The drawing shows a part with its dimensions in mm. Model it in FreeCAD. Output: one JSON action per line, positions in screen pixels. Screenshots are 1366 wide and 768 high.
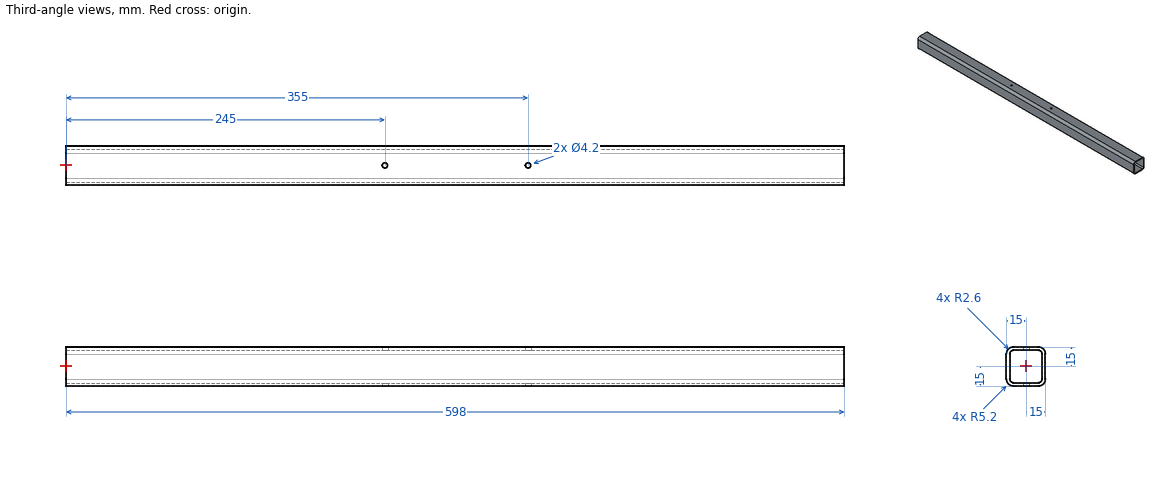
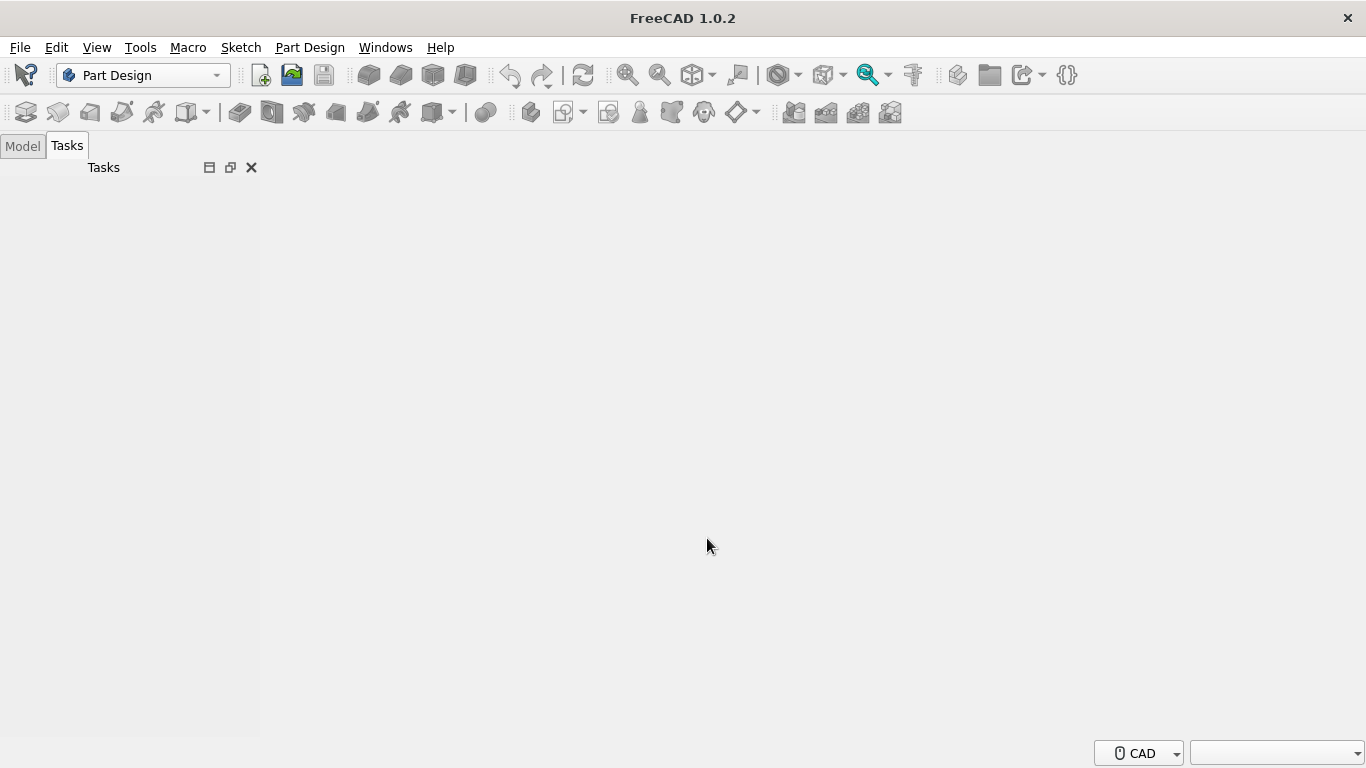
{"action": "left_click", "coordinate": [260, 76]}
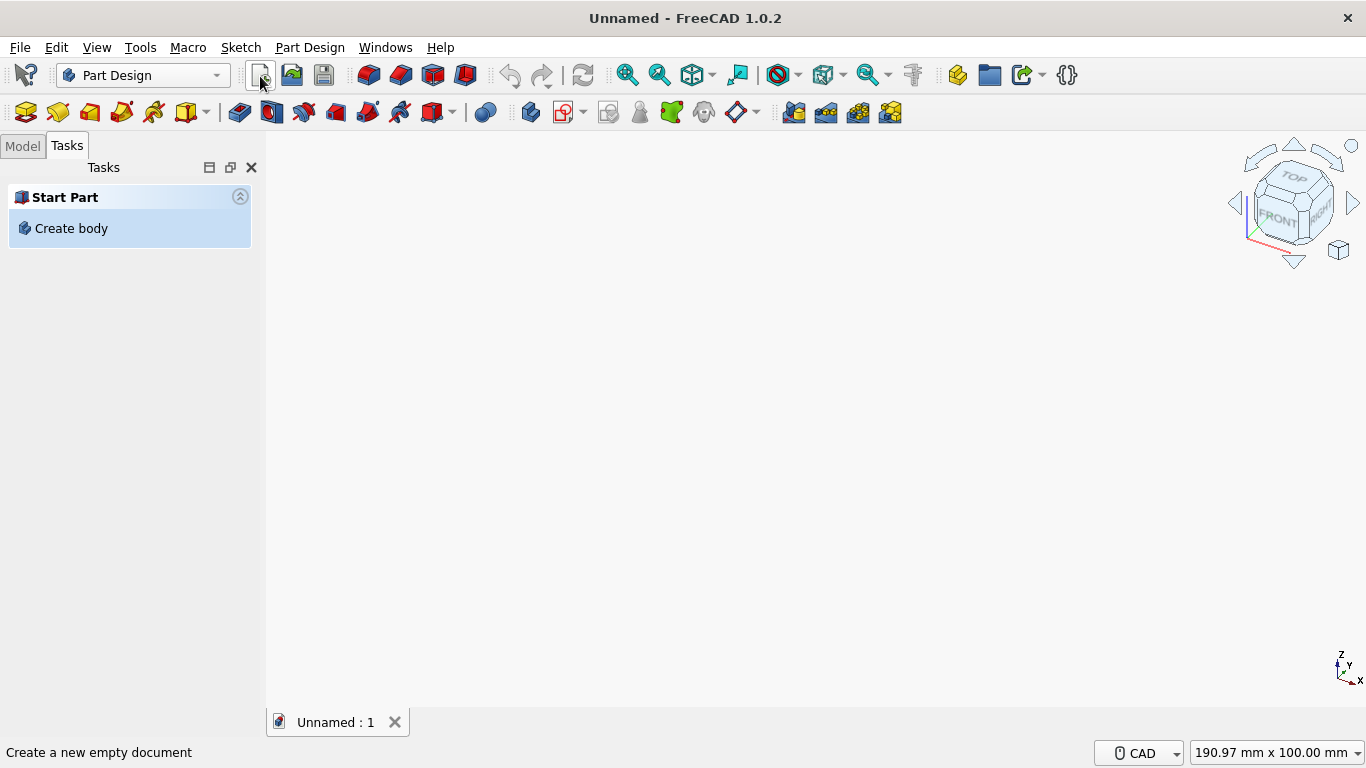
{"action": "left_click", "coordinate": [564, 112]}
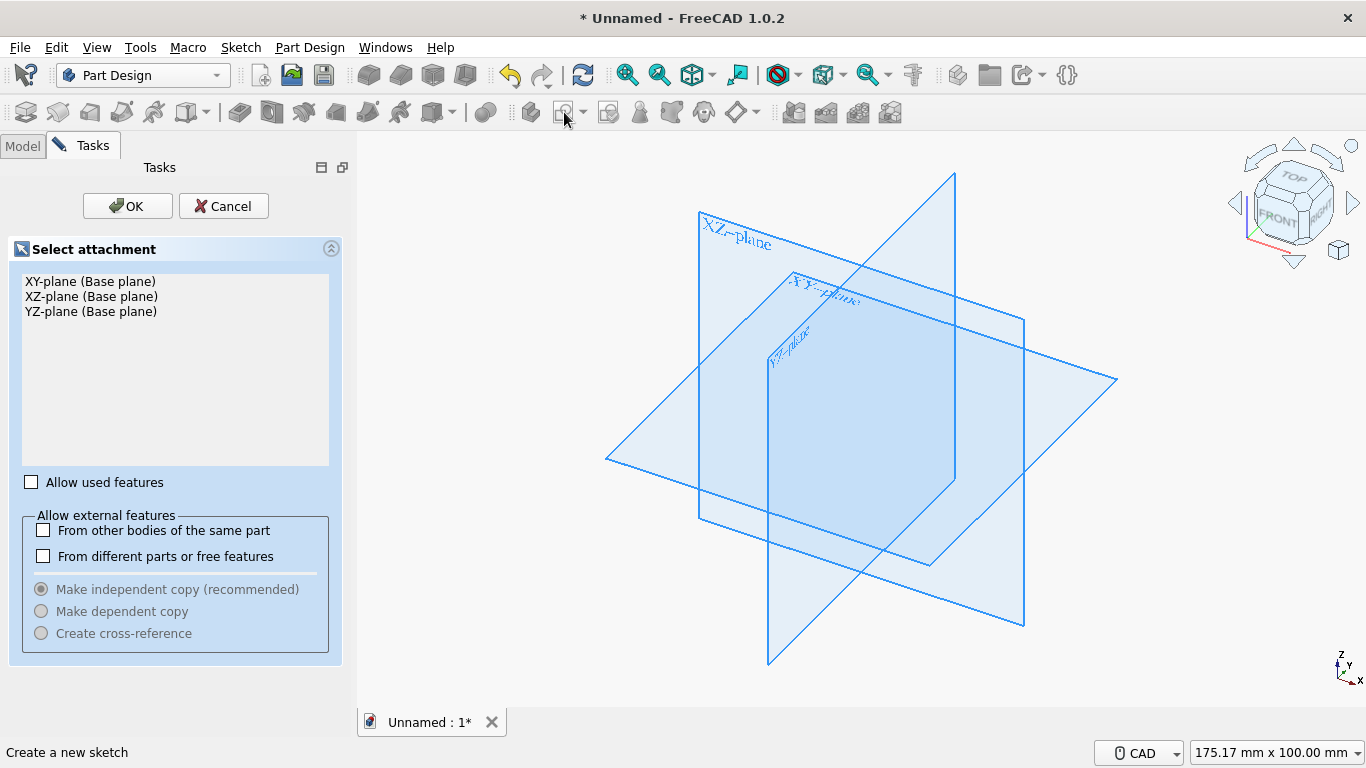
{"action": "left_click", "coordinate": [82, 312]}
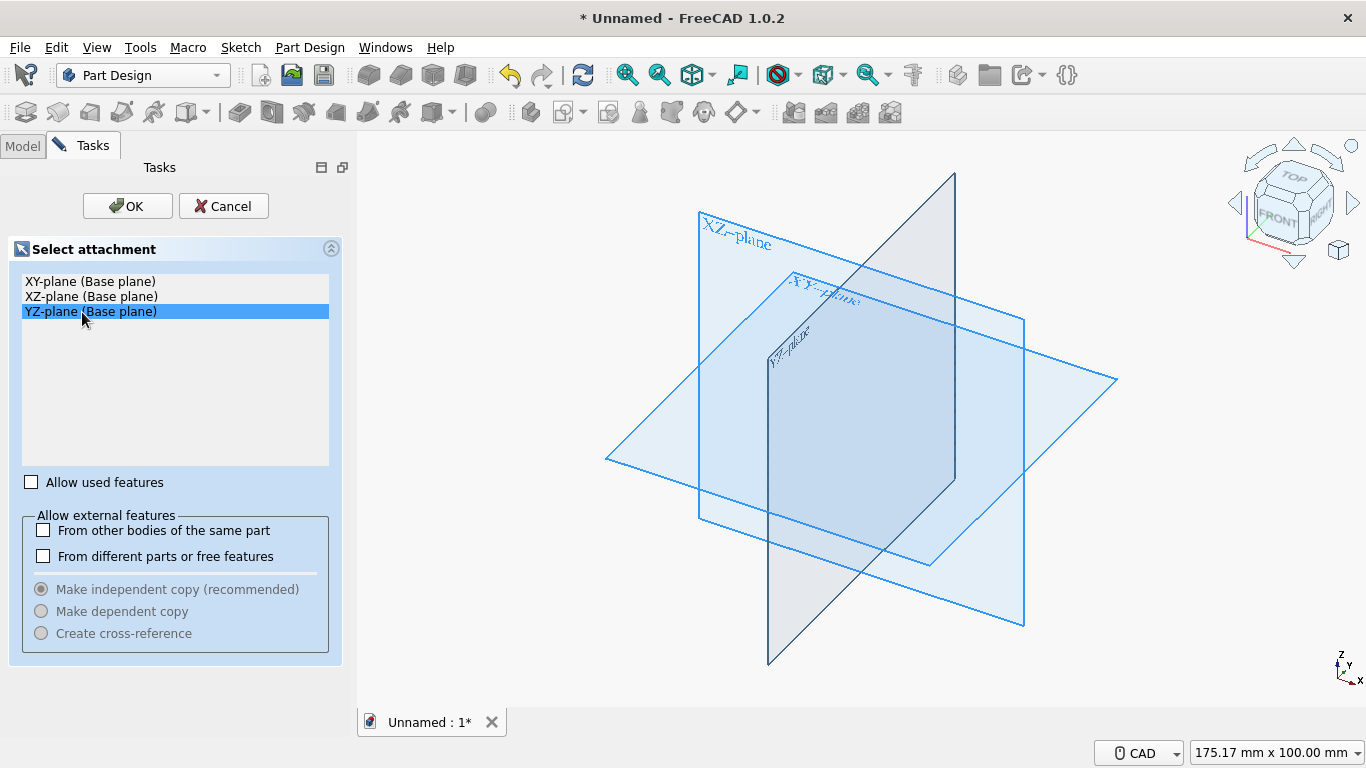
{"action": "left_click", "coordinate": [128, 206]}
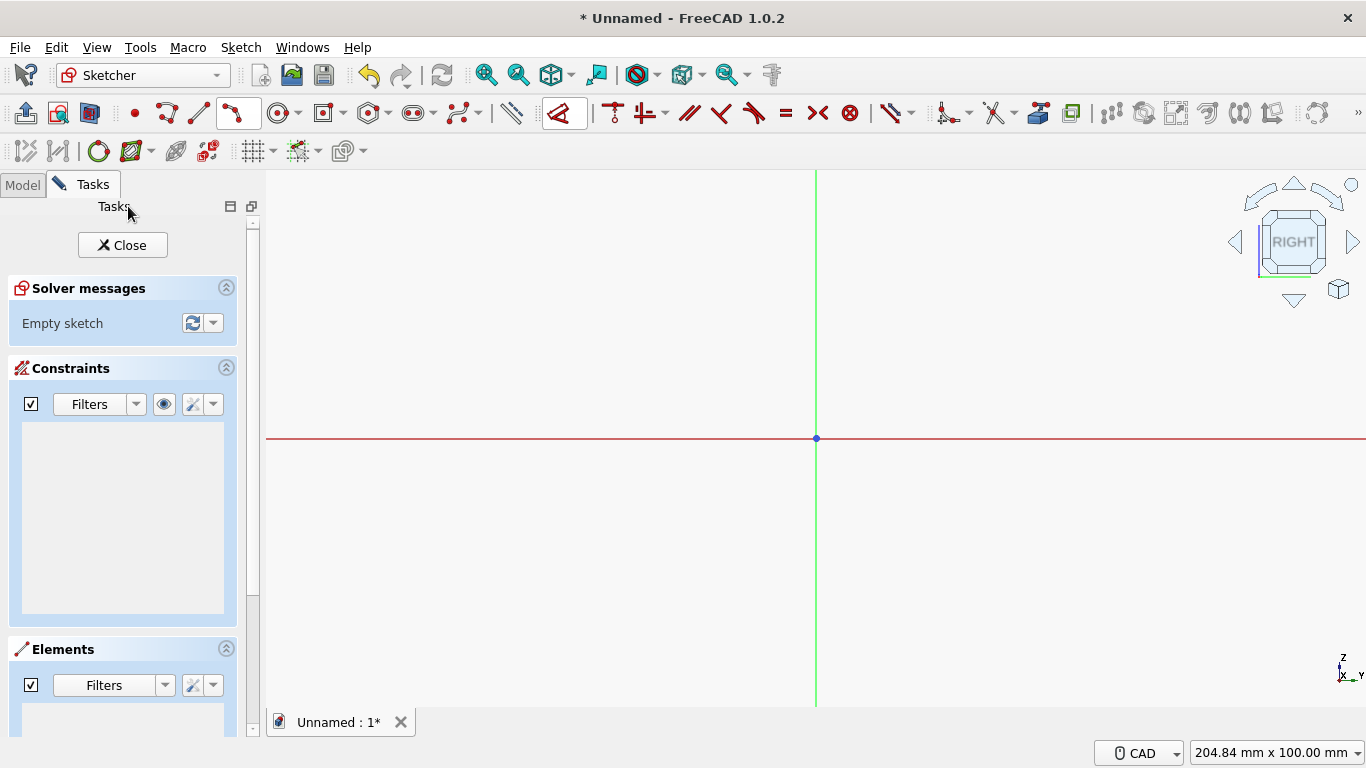
{"action": "scroll", "coordinate": [872, 438], "scroll_direction": "up", "scroll_amount": 4}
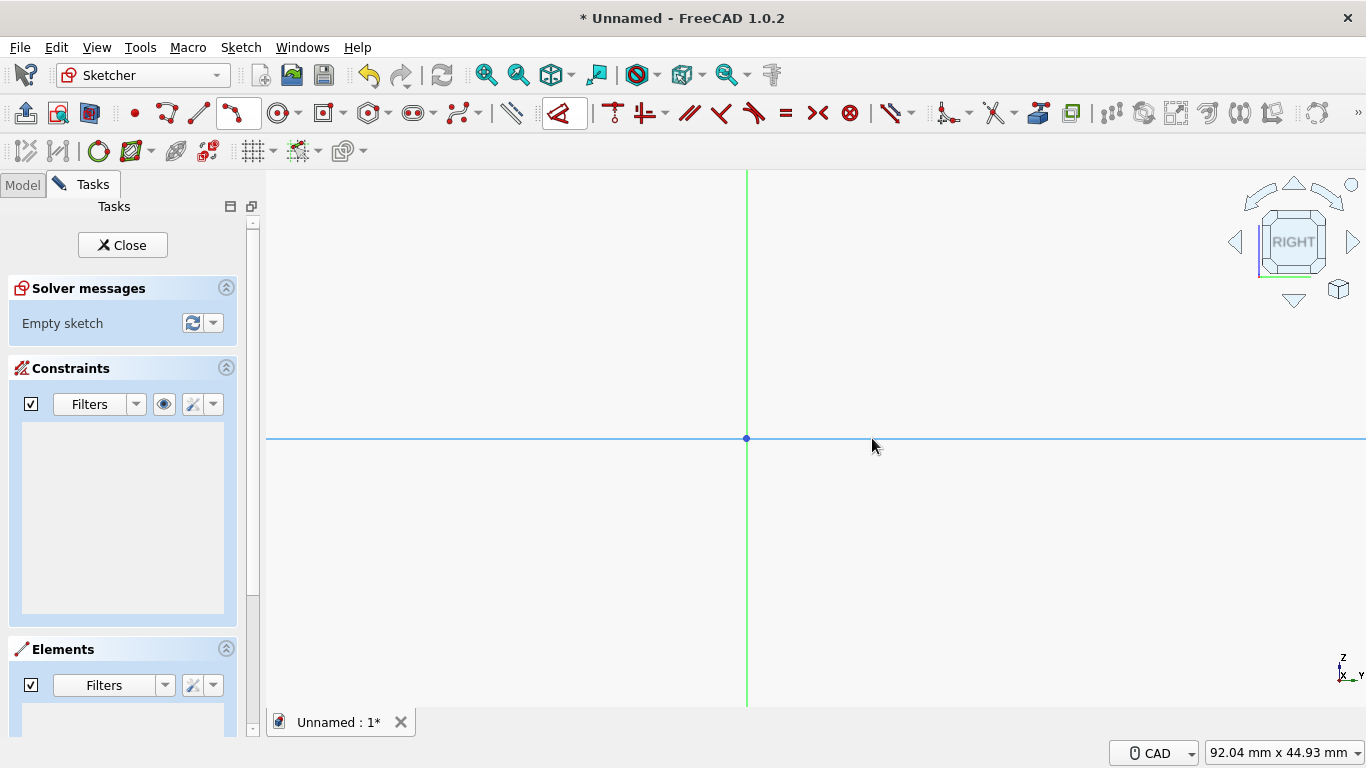
{"action": "key", "text": "g l"}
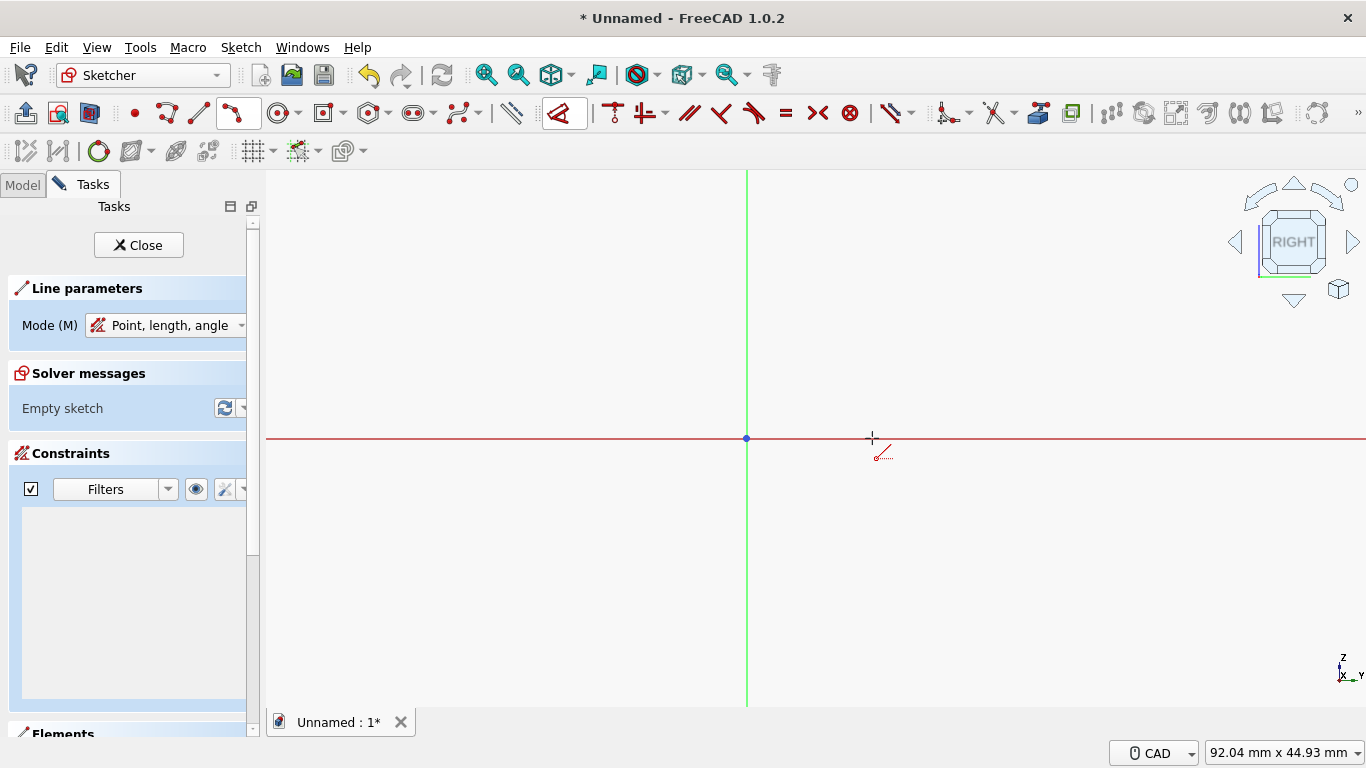
{"action": "left_click", "coordinate": [567, 321]}
{"action": "left_click", "coordinate": [567, 556]}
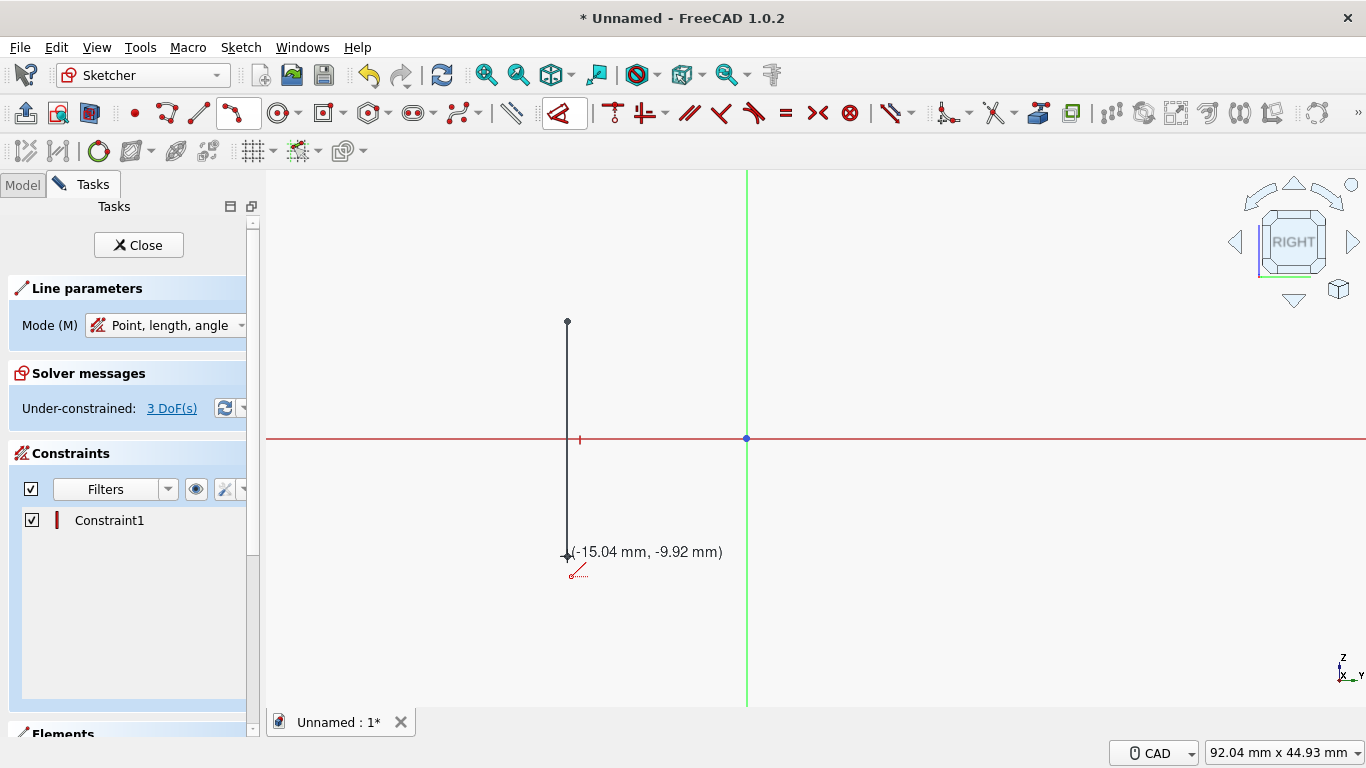
{"action": "left_click", "coordinate": [630, 618]}
{"action": "left_click", "coordinate": [864, 618]}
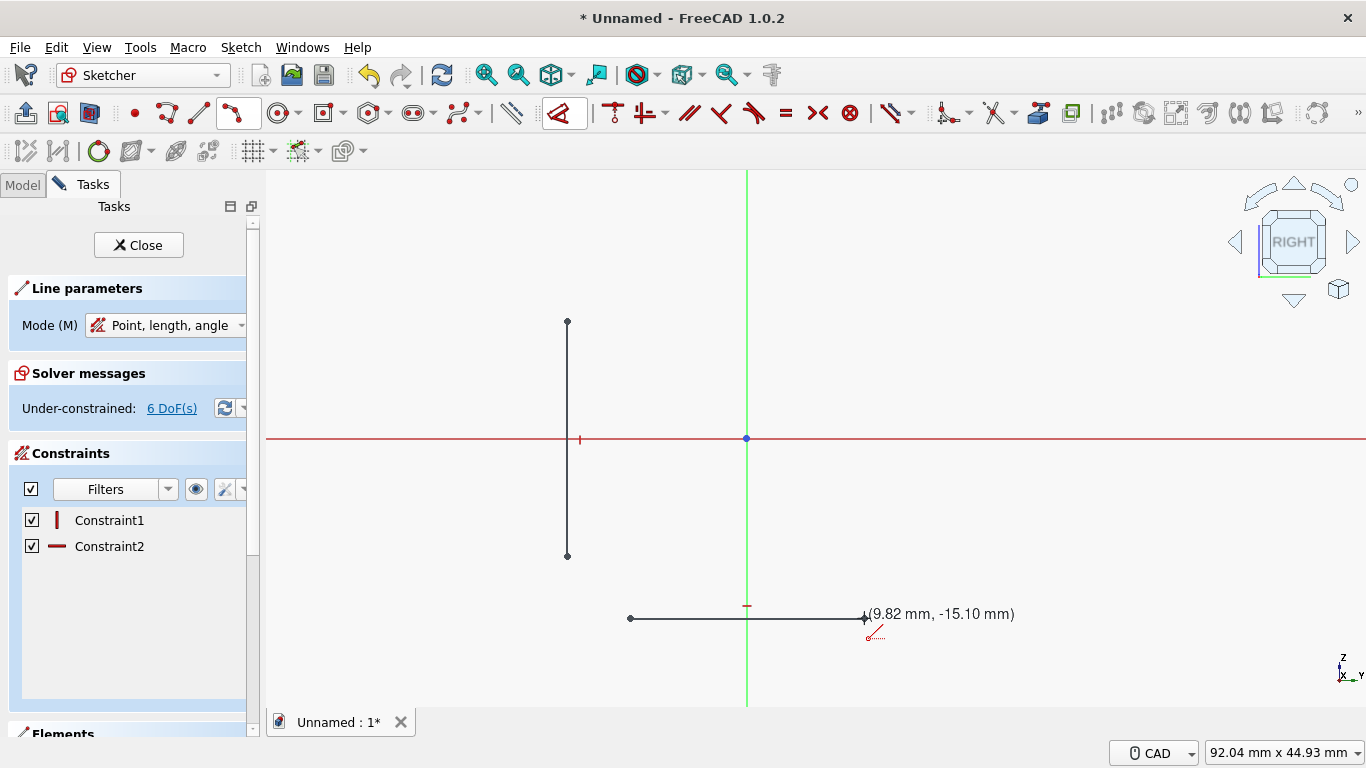
{"action": "left_click", "coordinate": [926, 556]}
{"action": "left_click", "coordinate": [926, 321]}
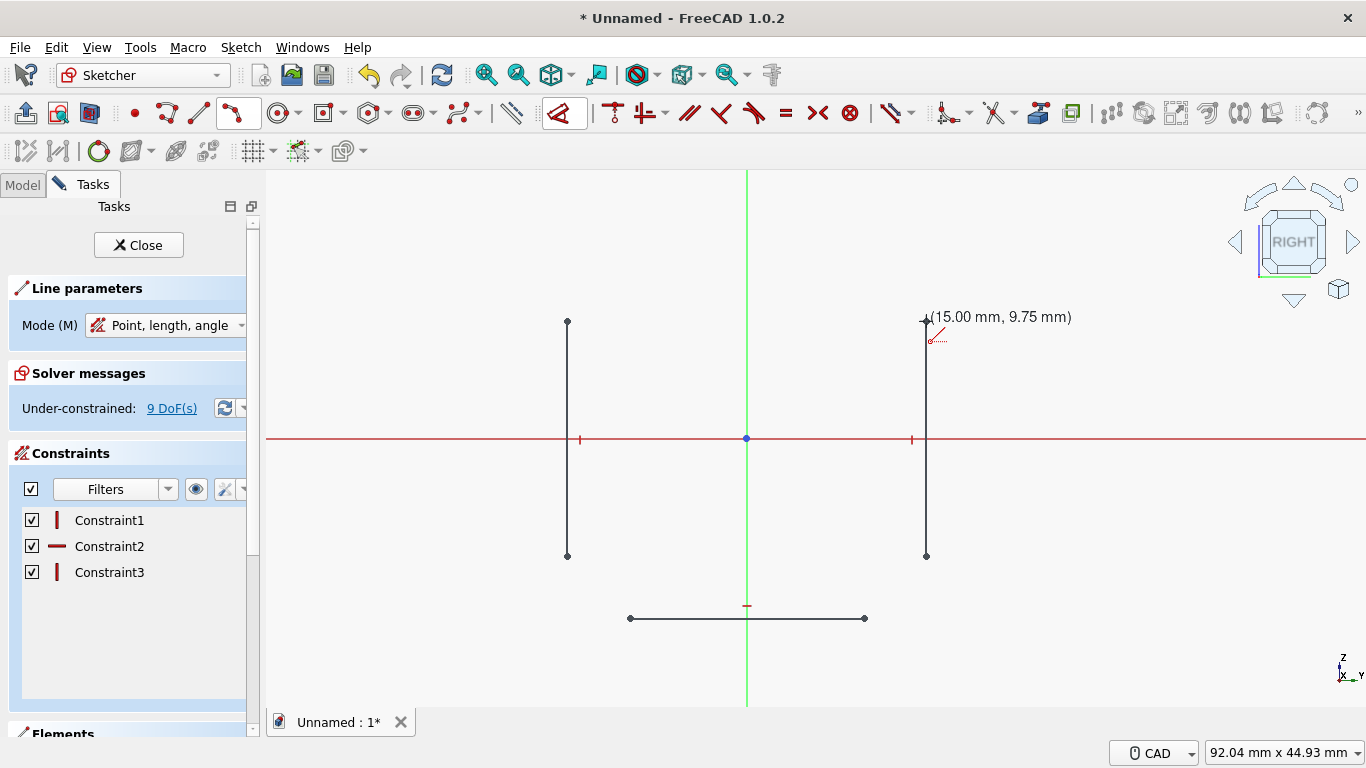
{"action": "left_click", "coordinate": [864, 259]}
{"action": "left_click", "coordinate": [630, 259]}